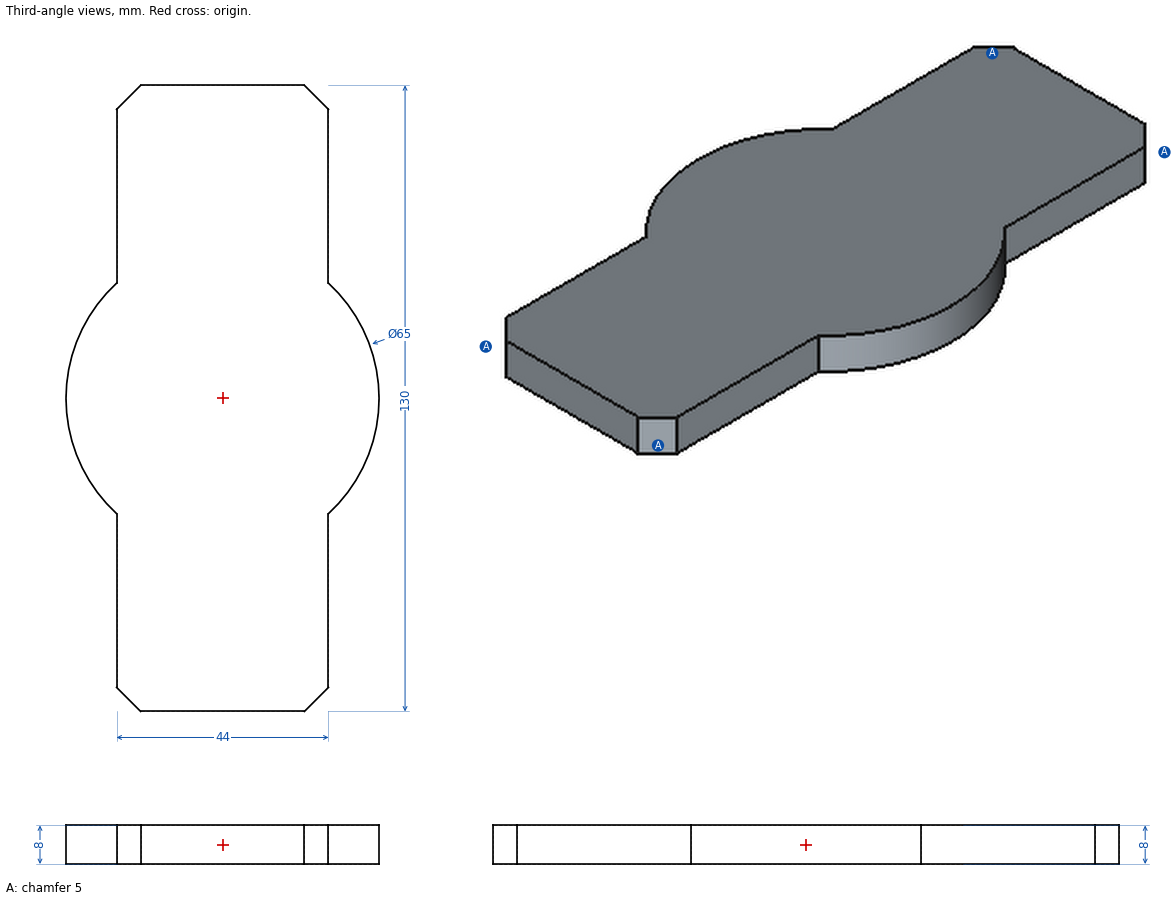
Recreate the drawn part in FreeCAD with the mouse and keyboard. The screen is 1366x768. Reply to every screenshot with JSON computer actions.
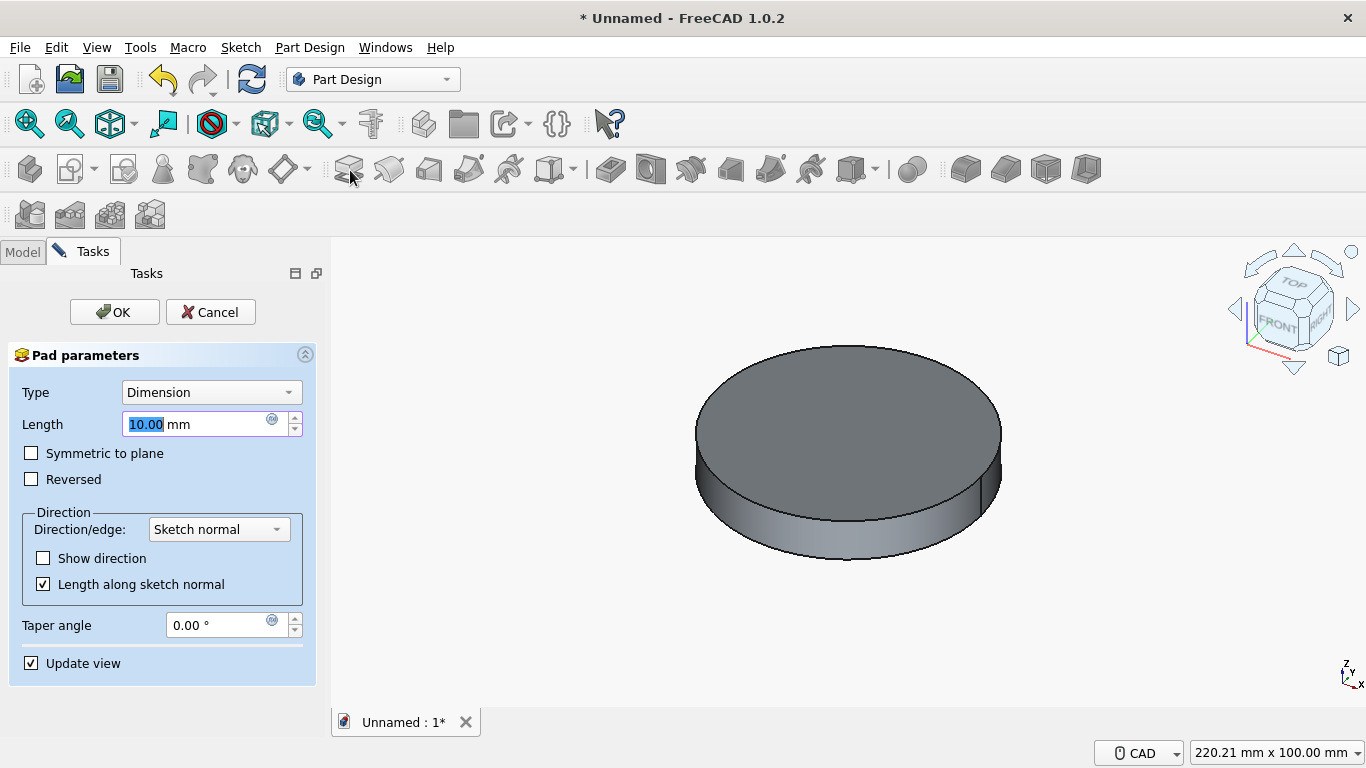
{"action": "type", "text": "8"}
{"action": "key", "text": "Tab"}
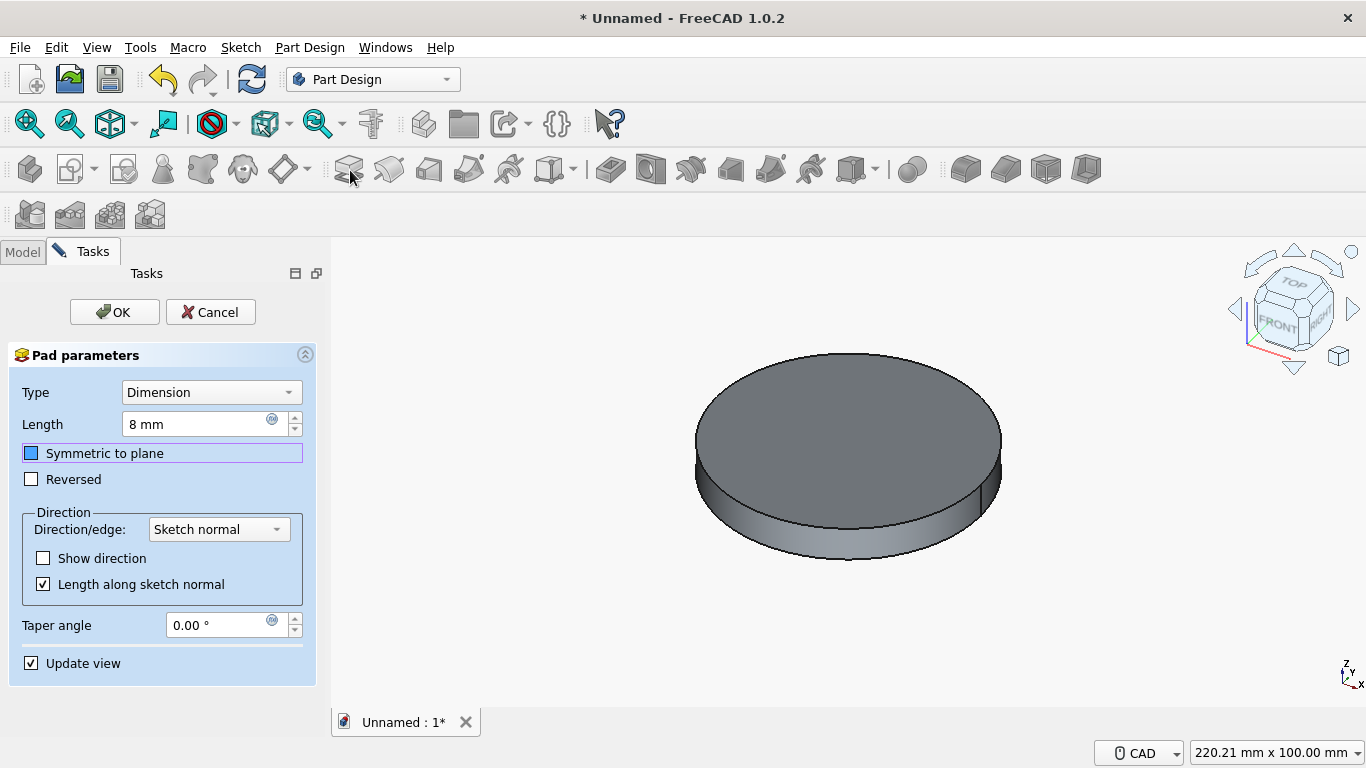
{"action": "left_click", "coordinate": [30, 453]}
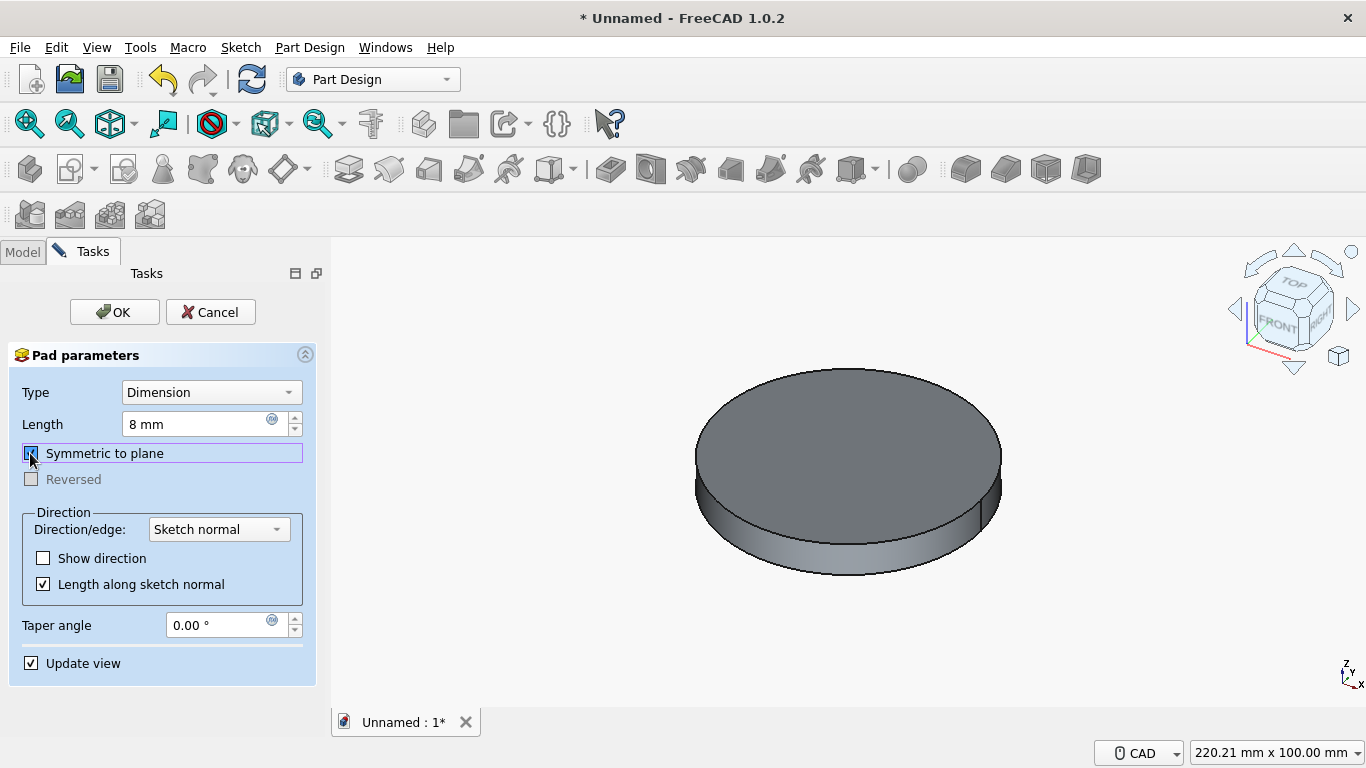
{"action": "left_click", "coordinate": [115, 312]}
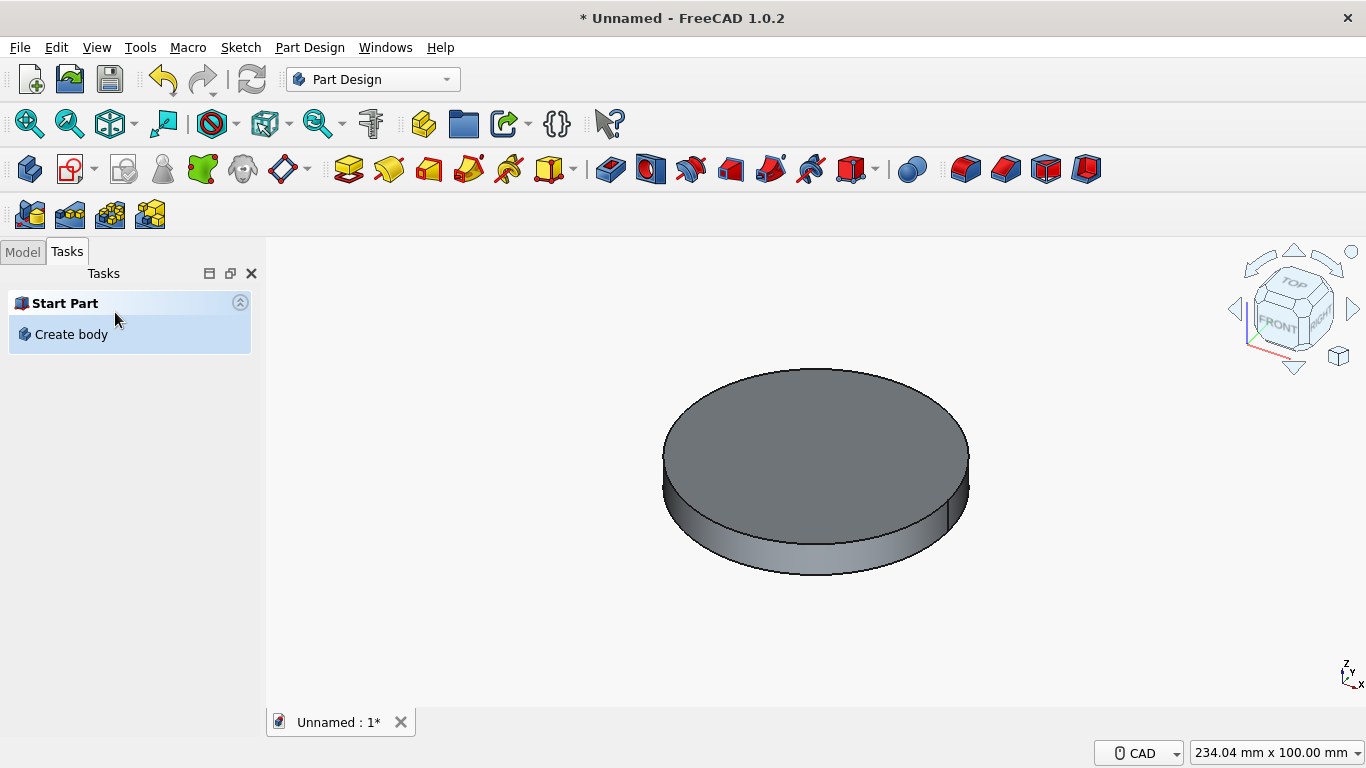
{"action": "left_click", "coordinate": [816, 456]}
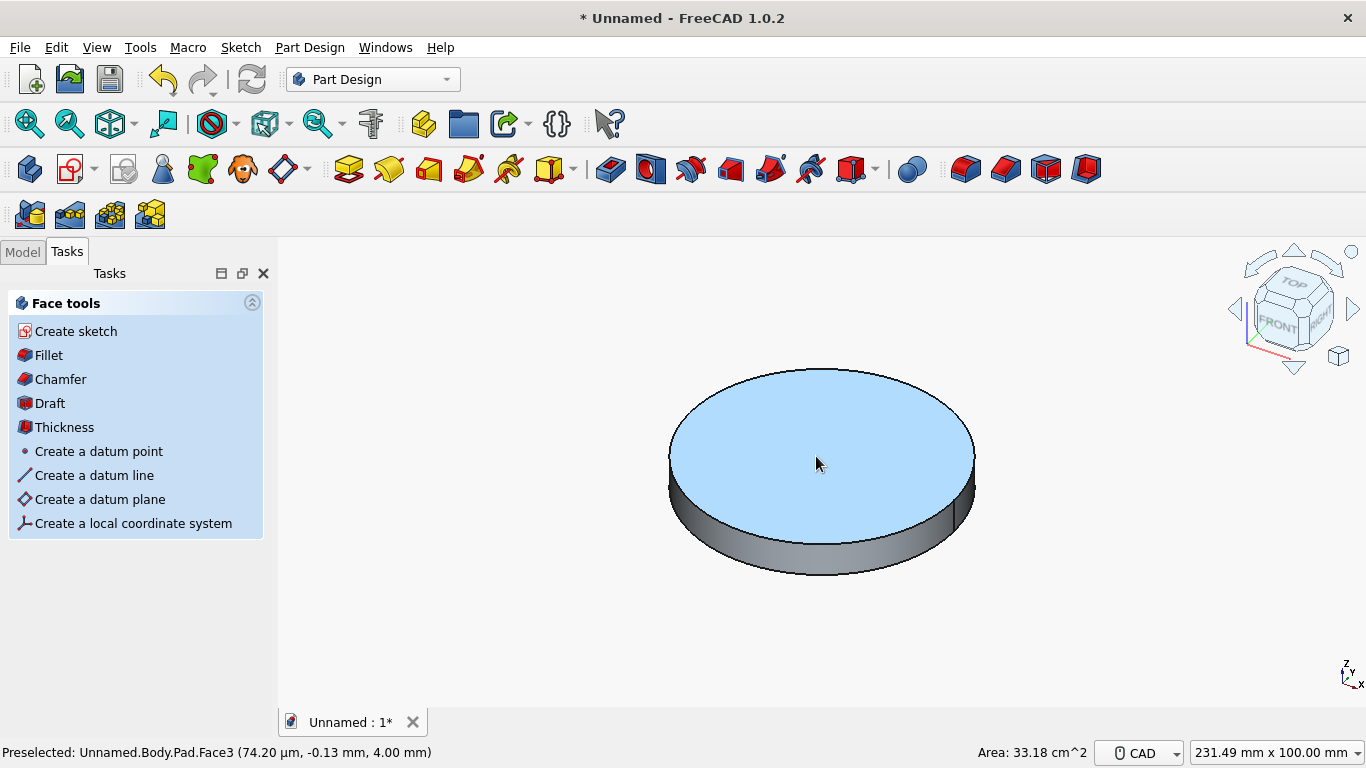
{"action": "left_click", "coordinate": [70, 170]}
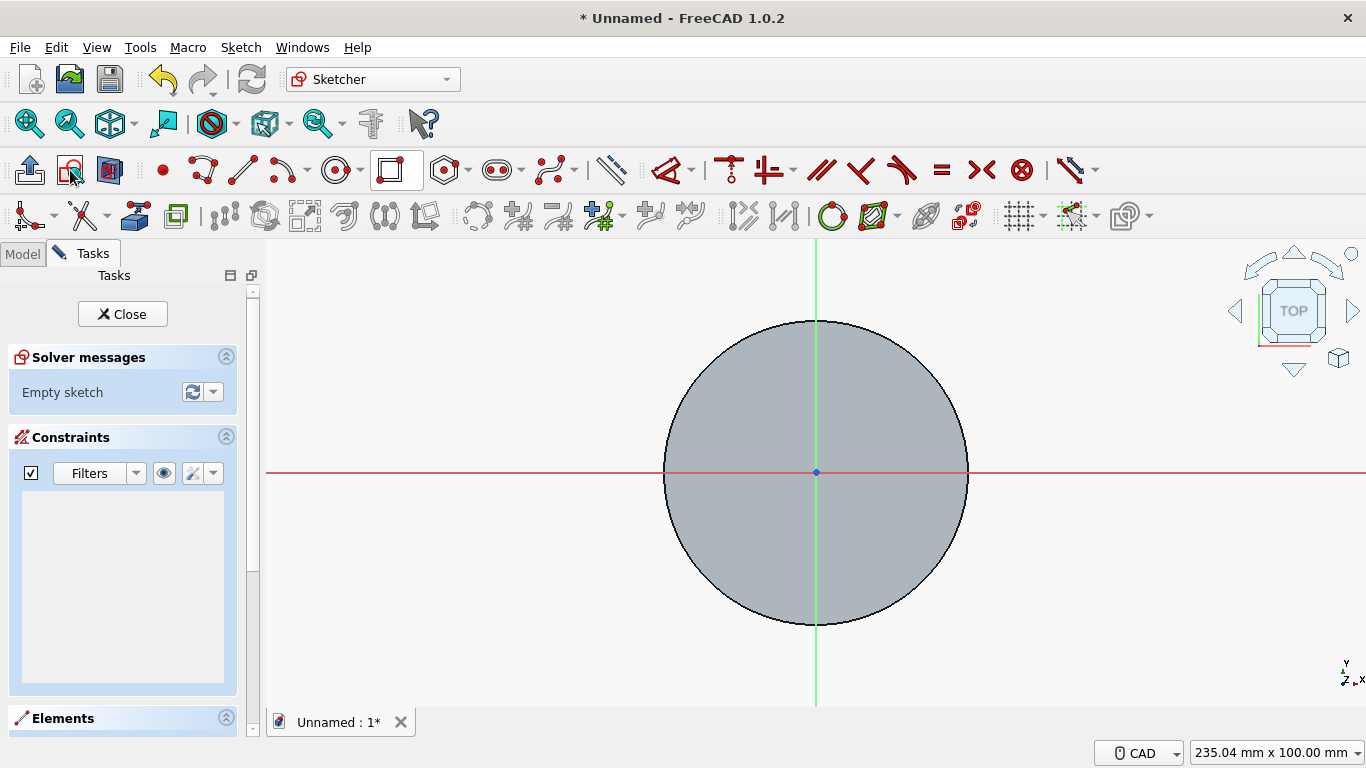
{"action": "scroll", "coordinate": [692, 473], "scroll_direction": "down", "scroll_amount": 4}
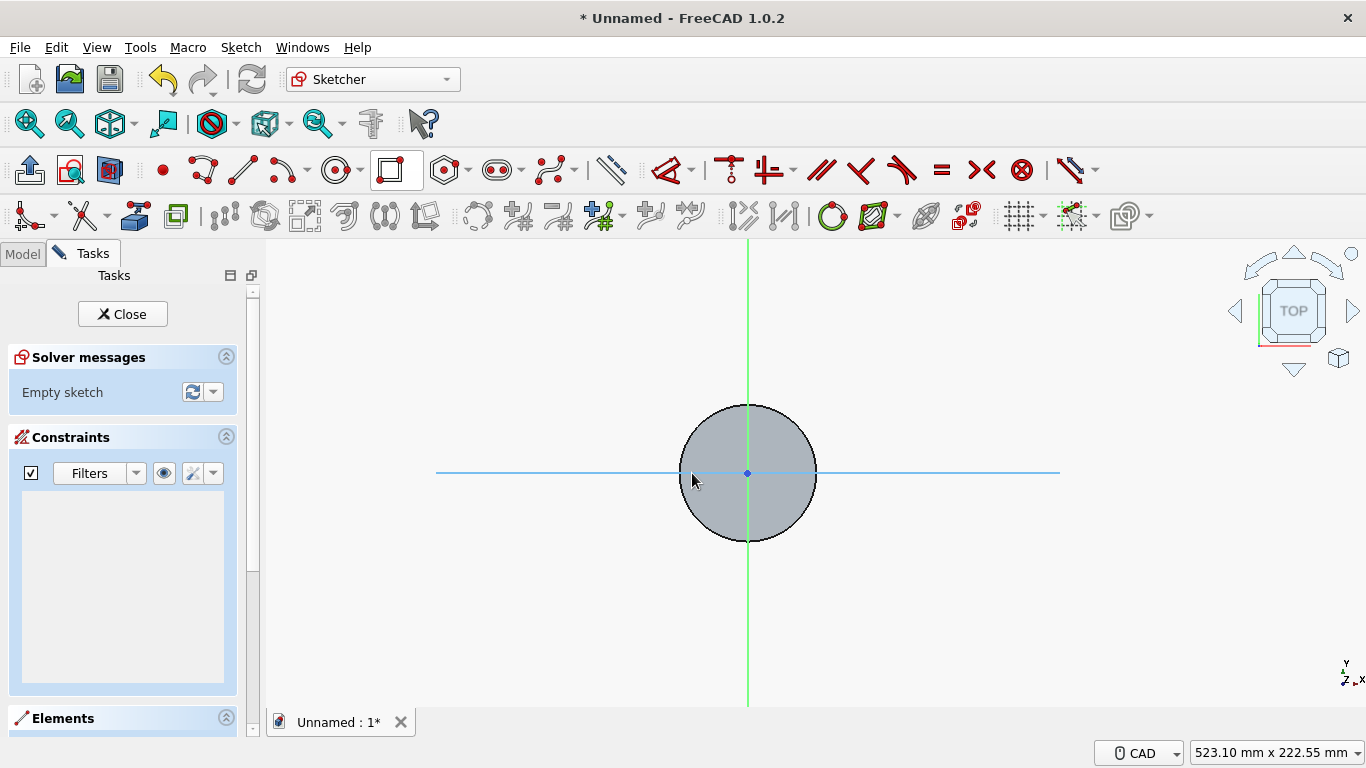
{"action": "left_click", "coordinate": [418, 170]}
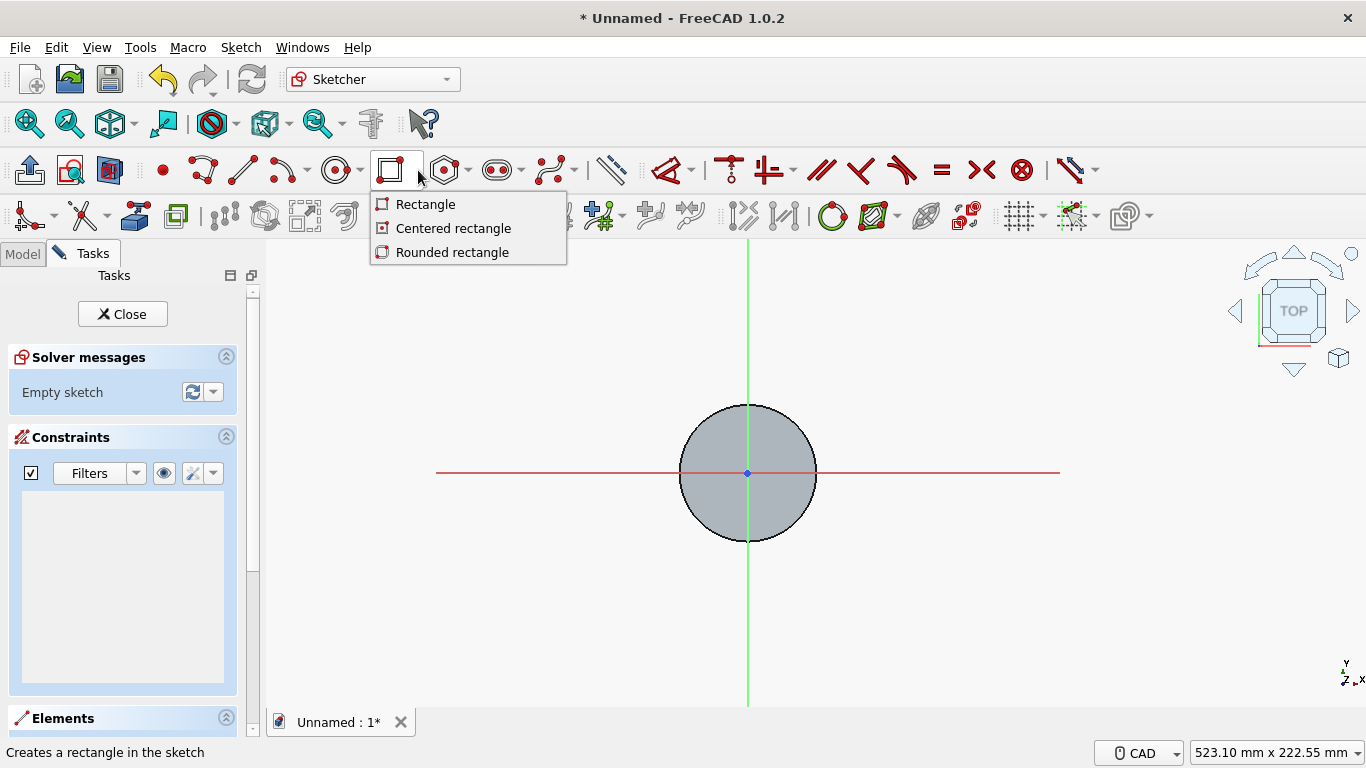
{"action": "left_click", "coordinate": [468, 228]}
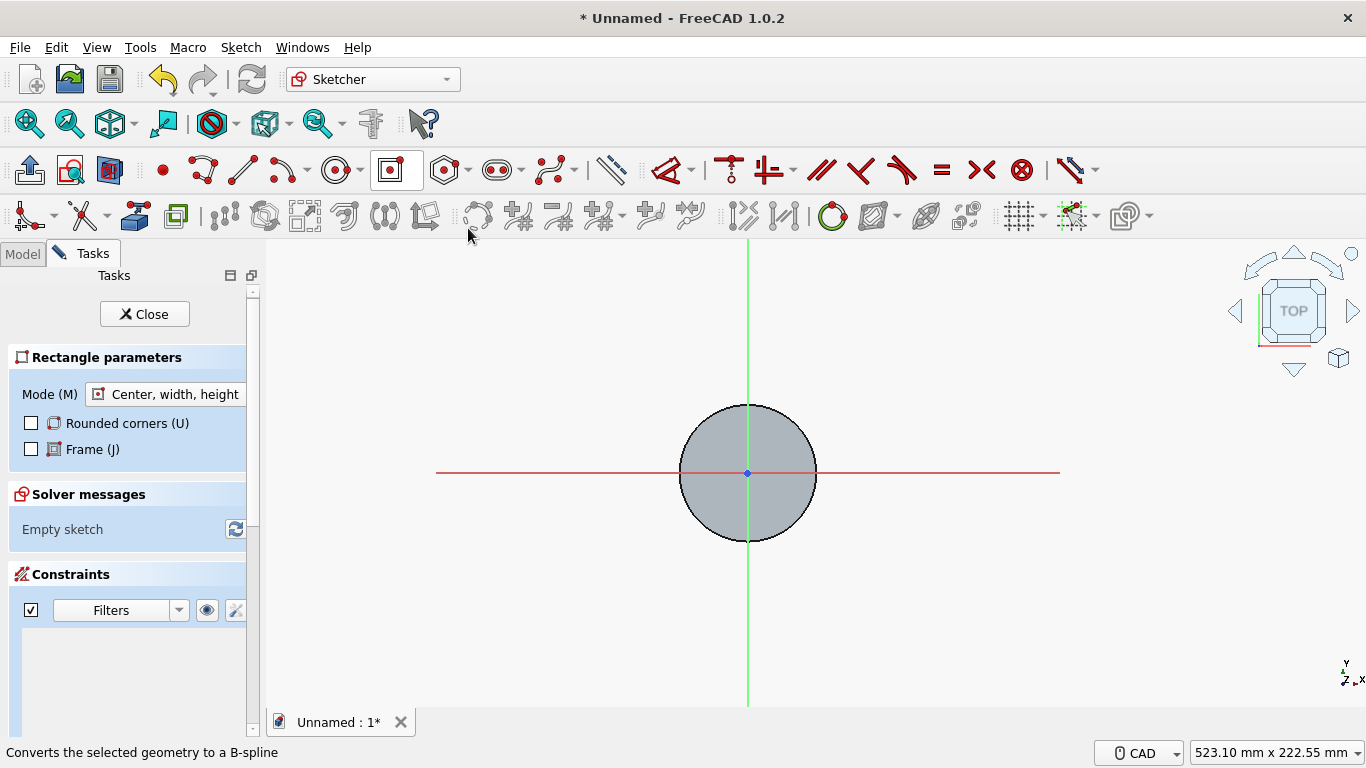
{"action": "left_click", "coordinate": [748, 473]}
{"action": "mouse_move", "coordinate": [794, 337]}